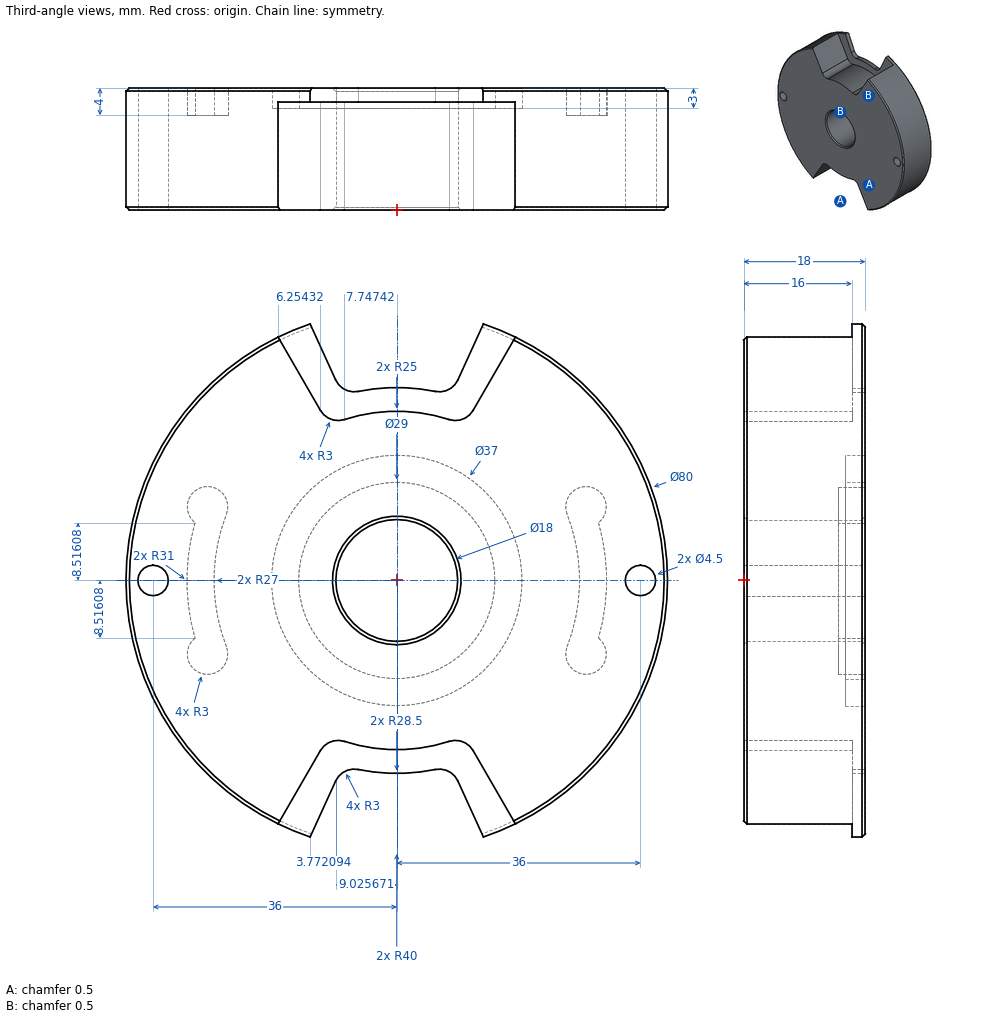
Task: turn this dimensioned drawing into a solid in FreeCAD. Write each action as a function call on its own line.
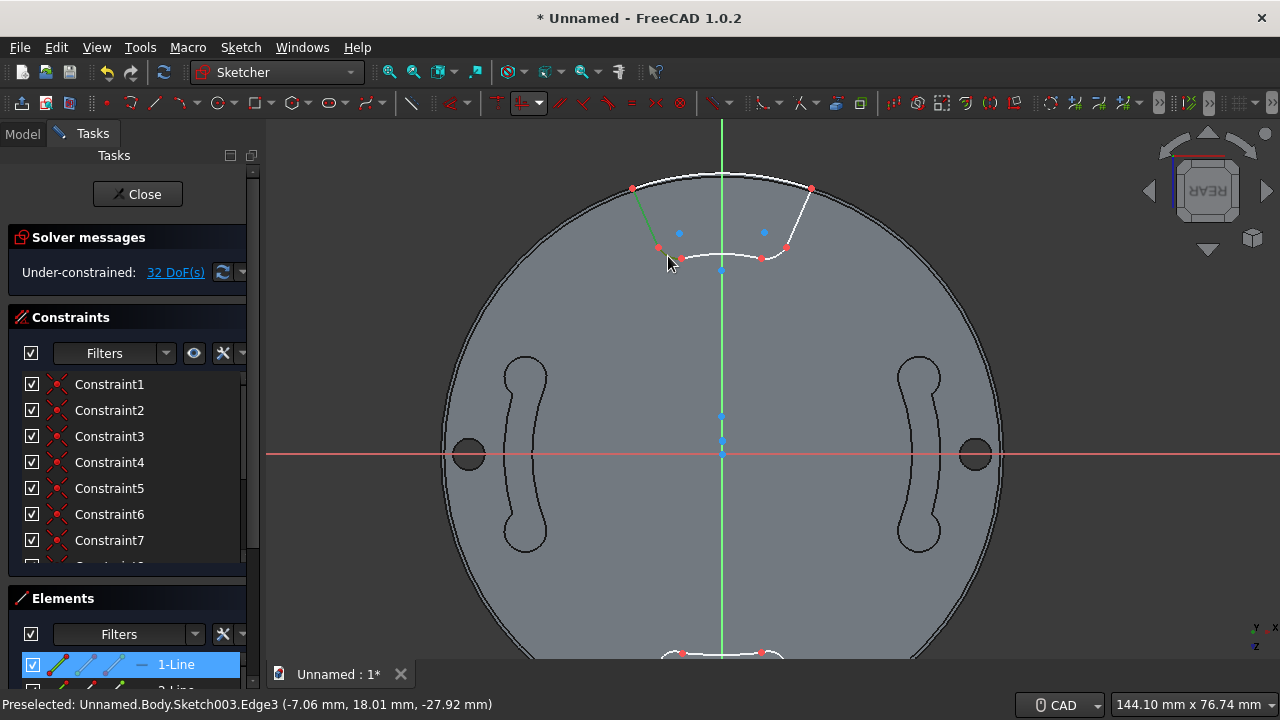
click(608, 104)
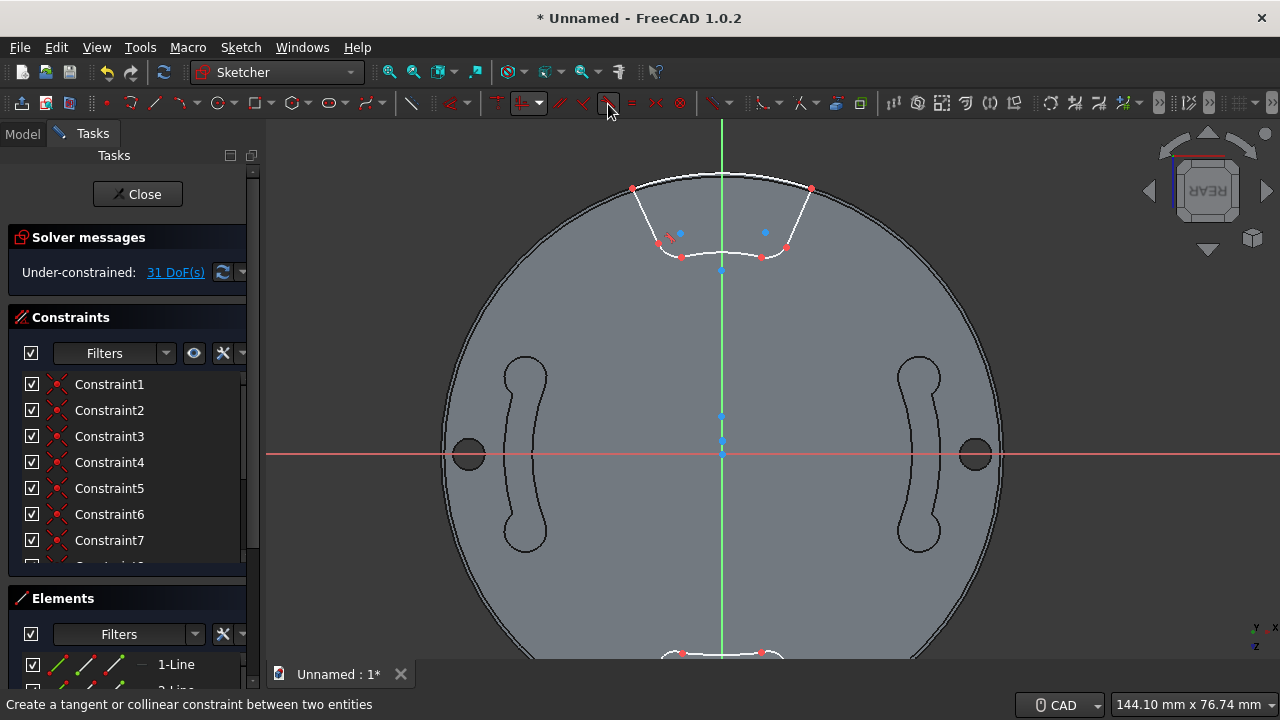
click(794, 230)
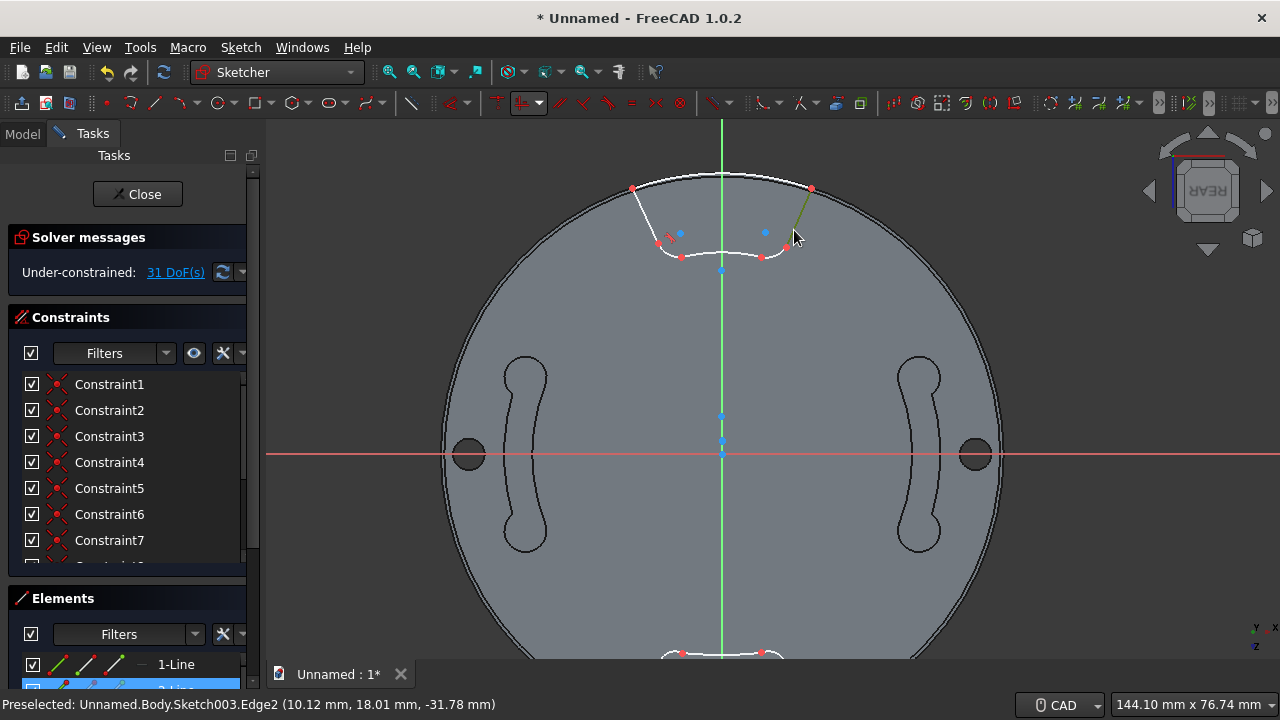
click(776, 256)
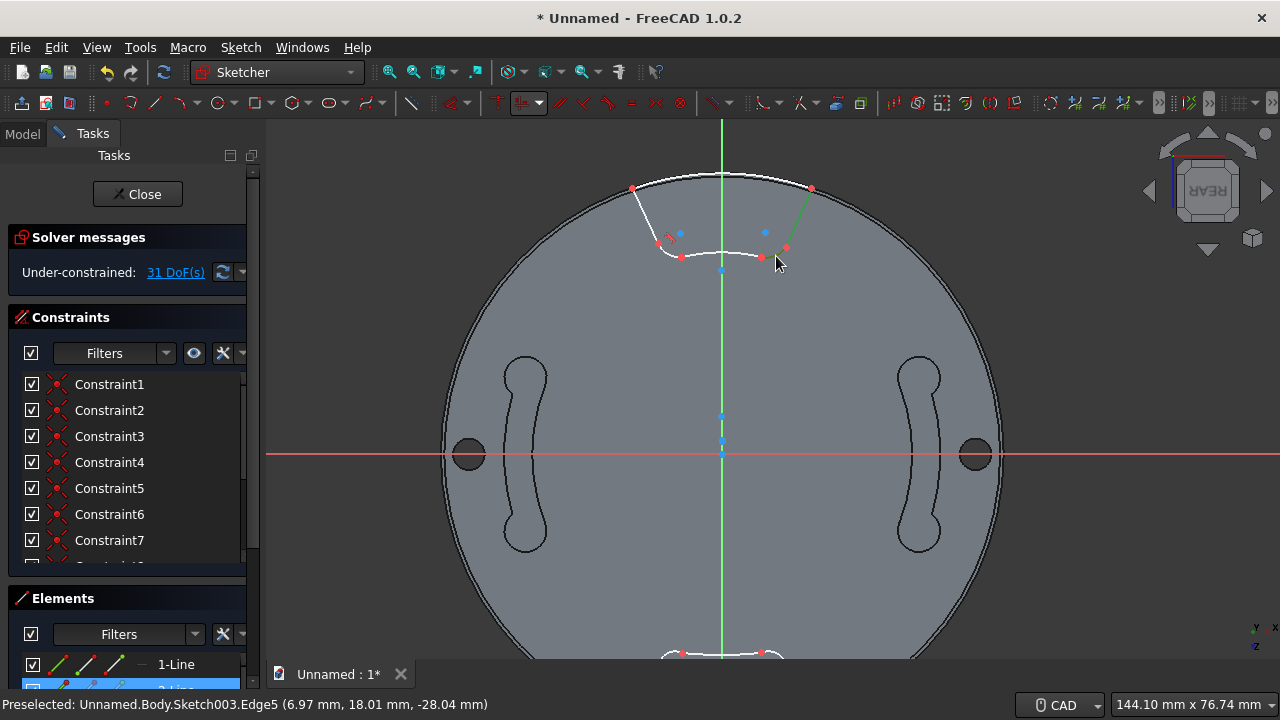
click(608, 104)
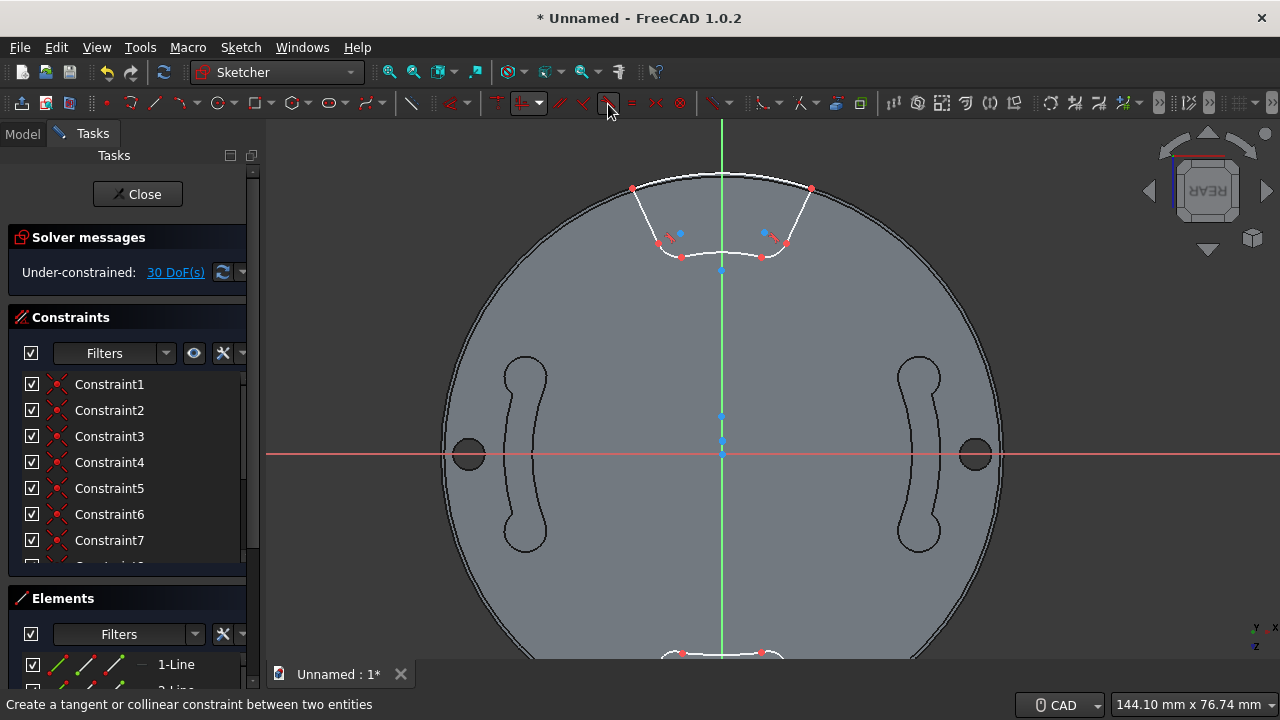
click(668, 254)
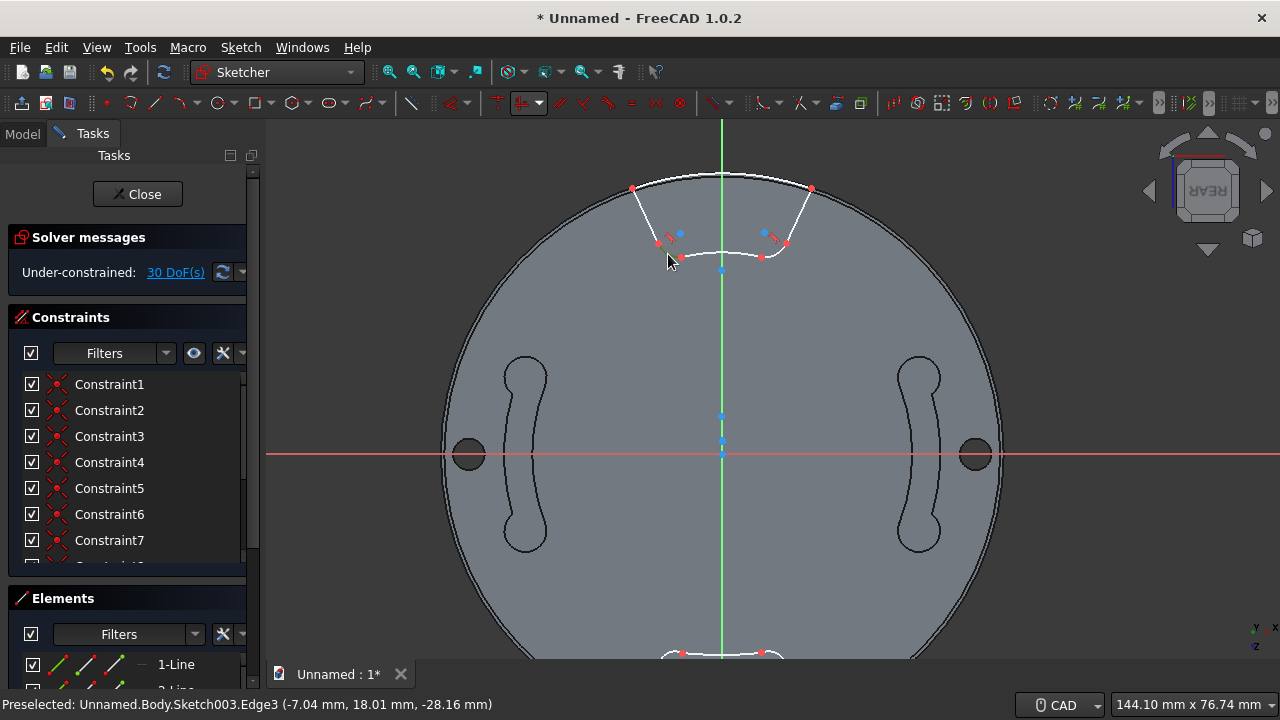
click(738, 253)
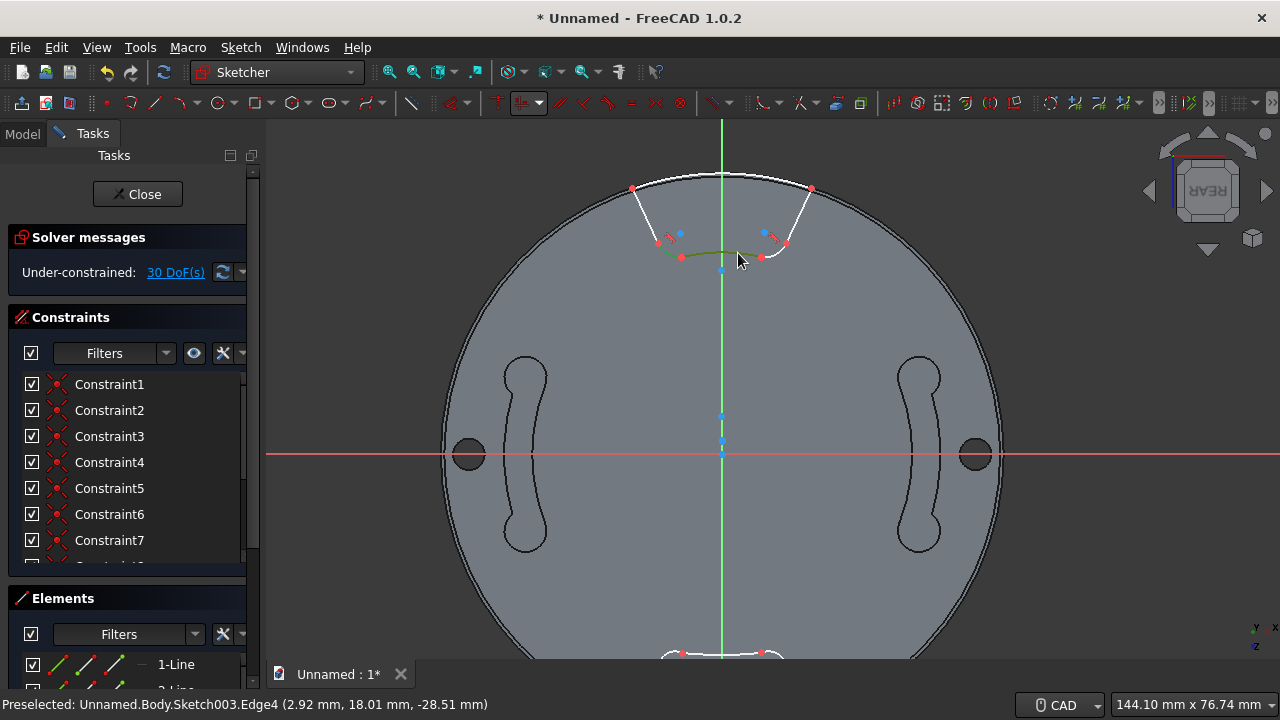
click(608, 104)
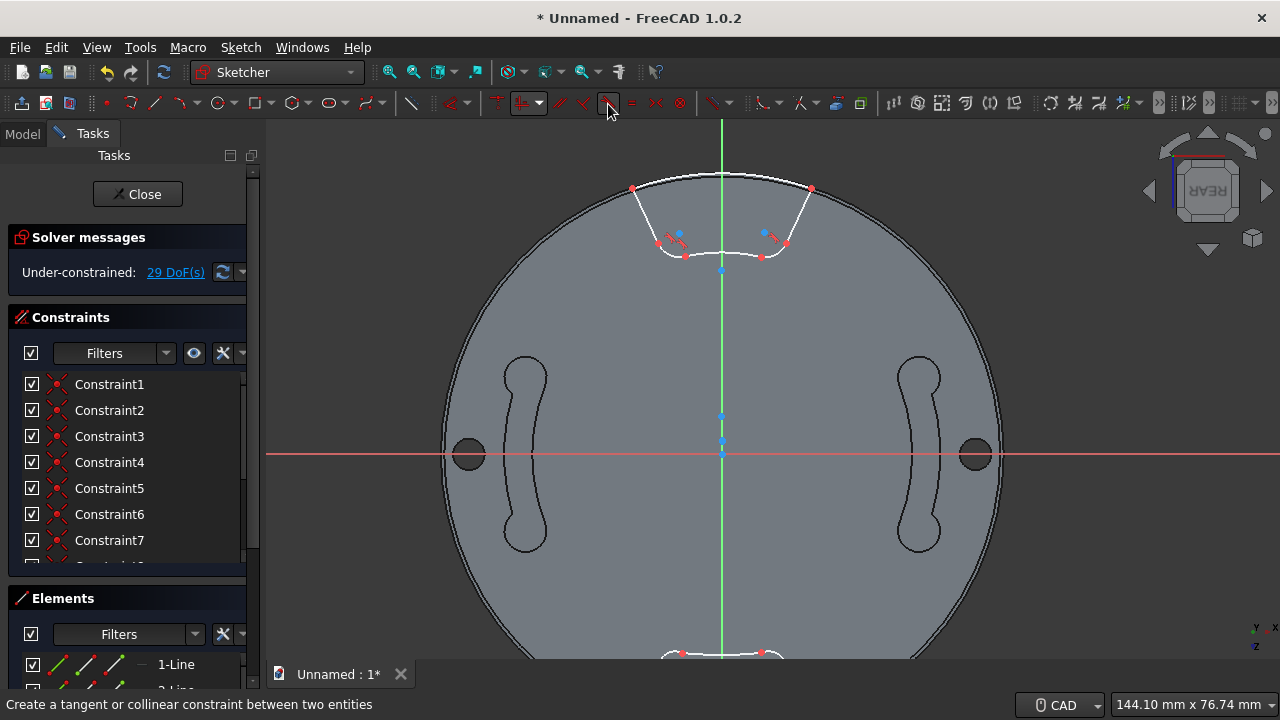
click(739, 253)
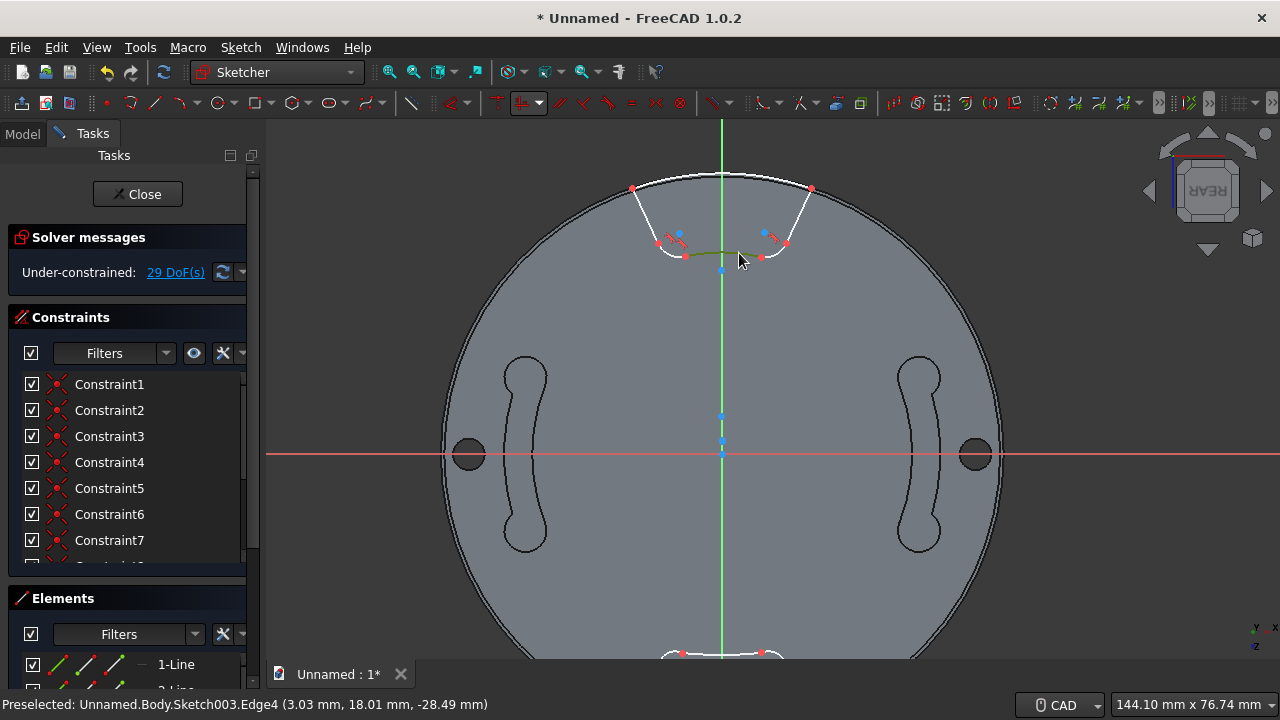
scroll(771, 257, up, 3)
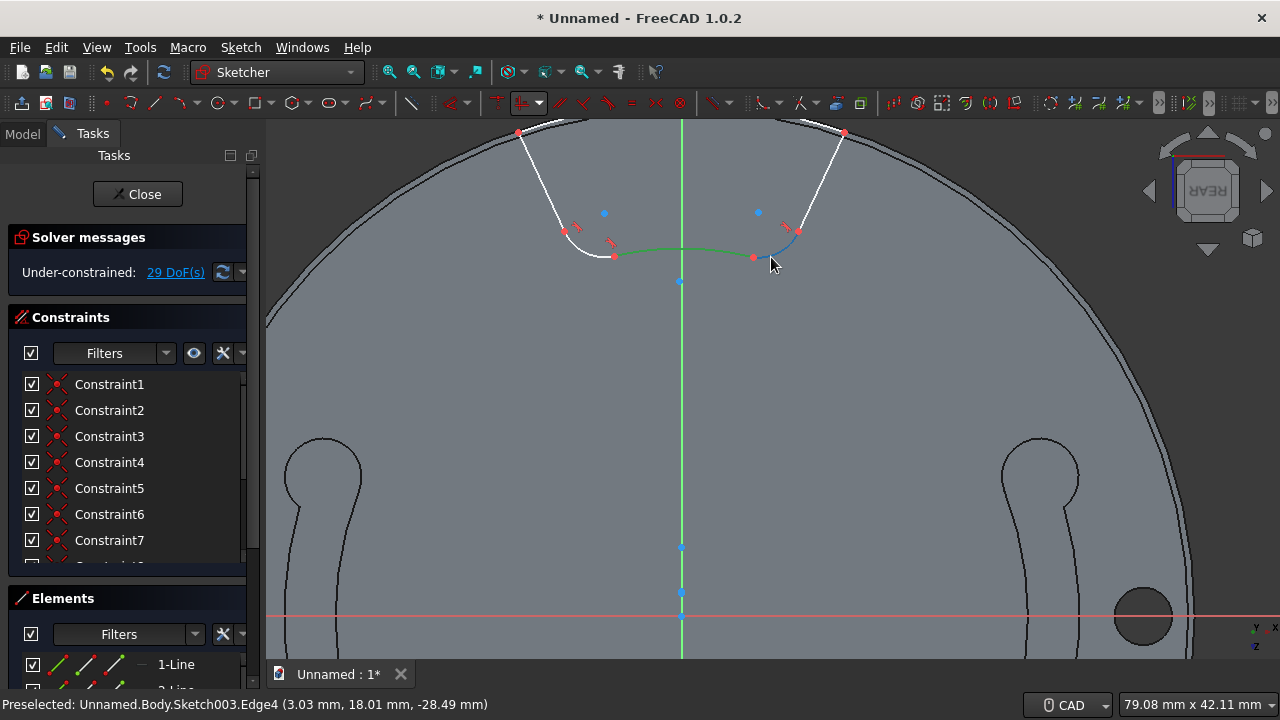
click(770, 256)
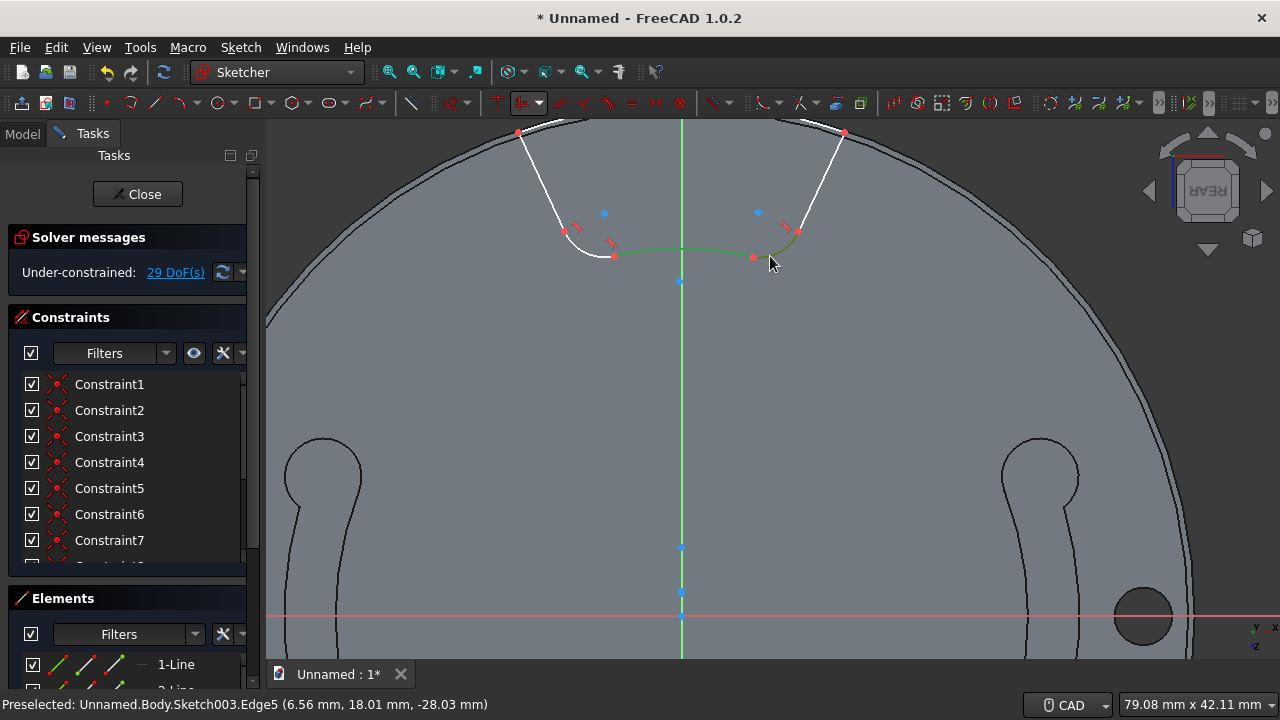
click(608, 104)